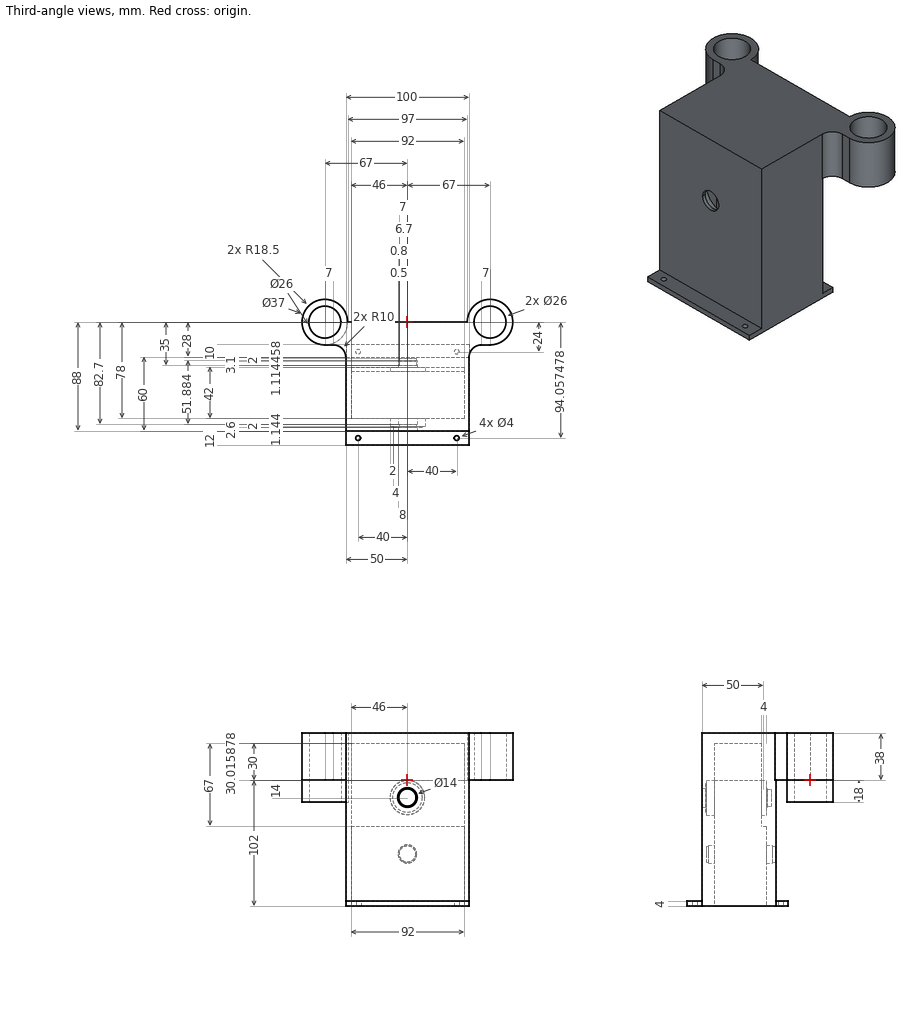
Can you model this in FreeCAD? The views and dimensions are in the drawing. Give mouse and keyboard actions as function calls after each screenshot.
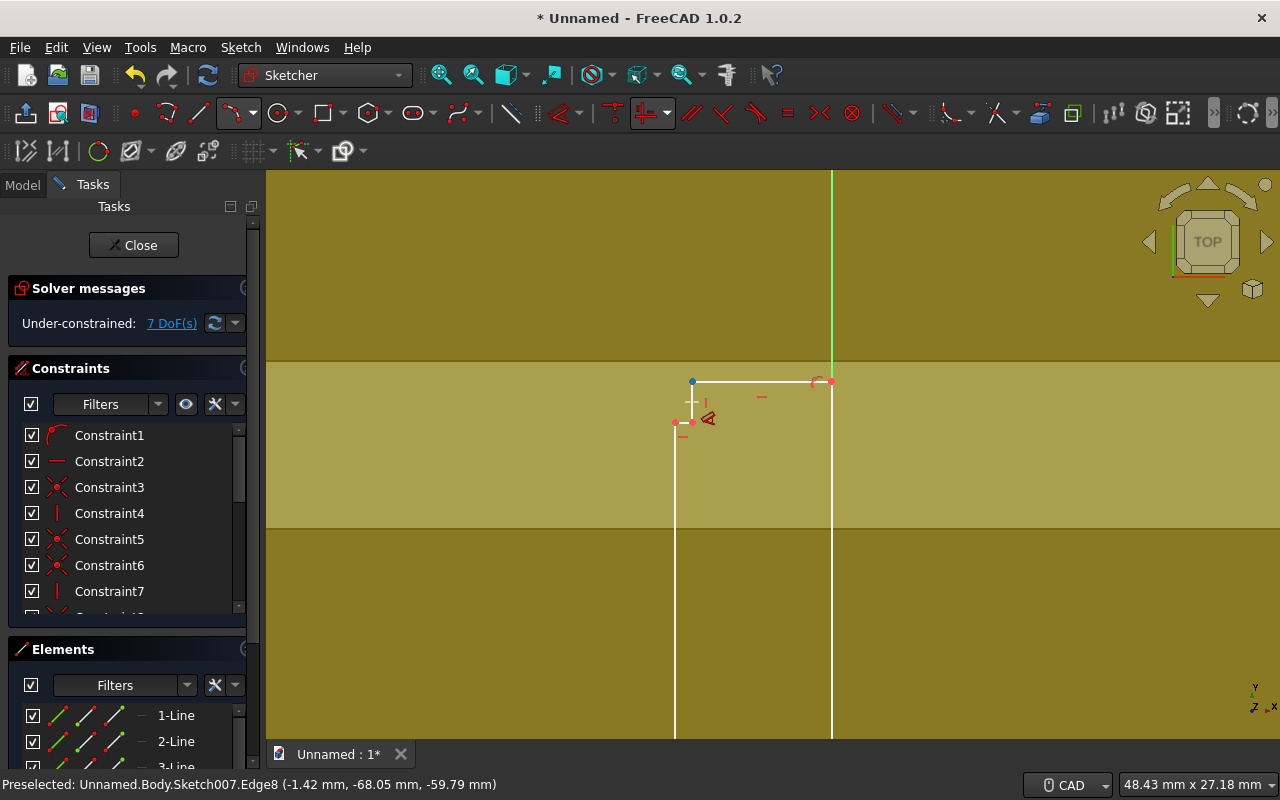
click(692, 402)
click(658, 402)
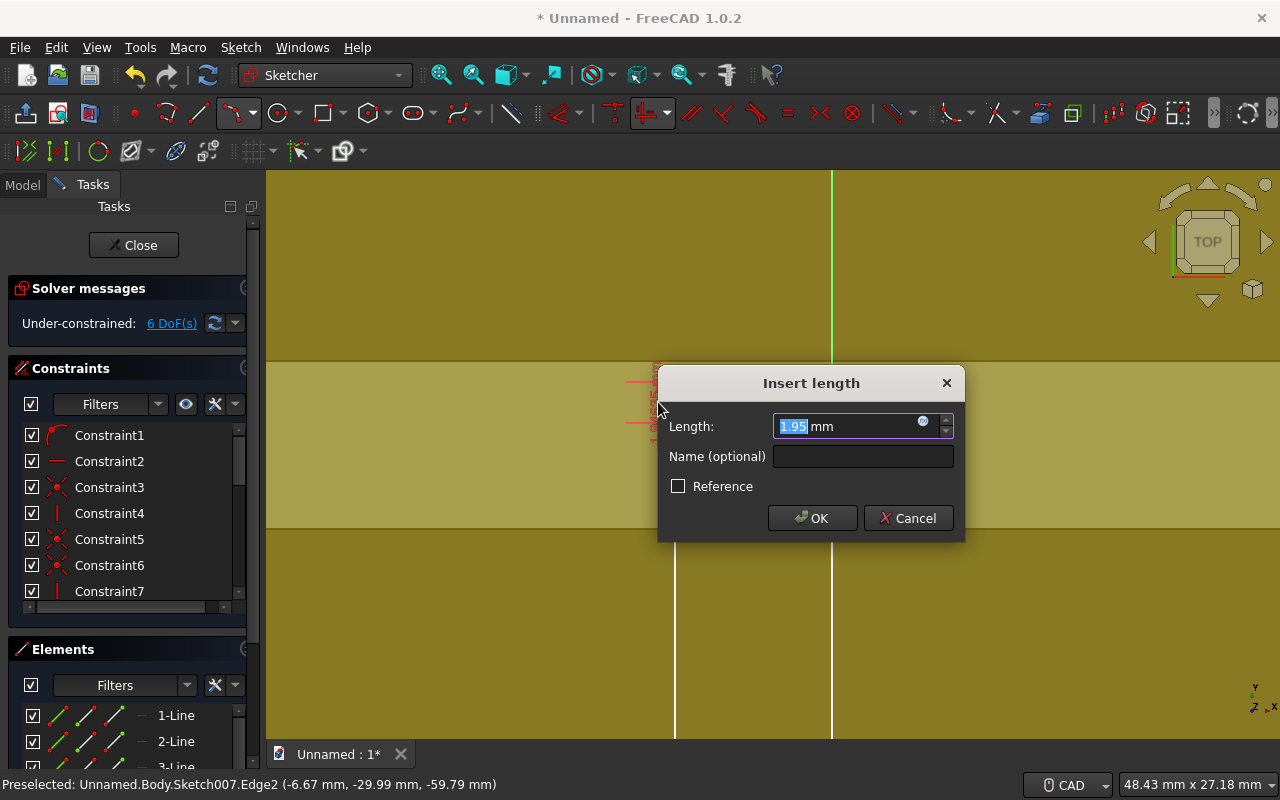
text(2)
key(Return)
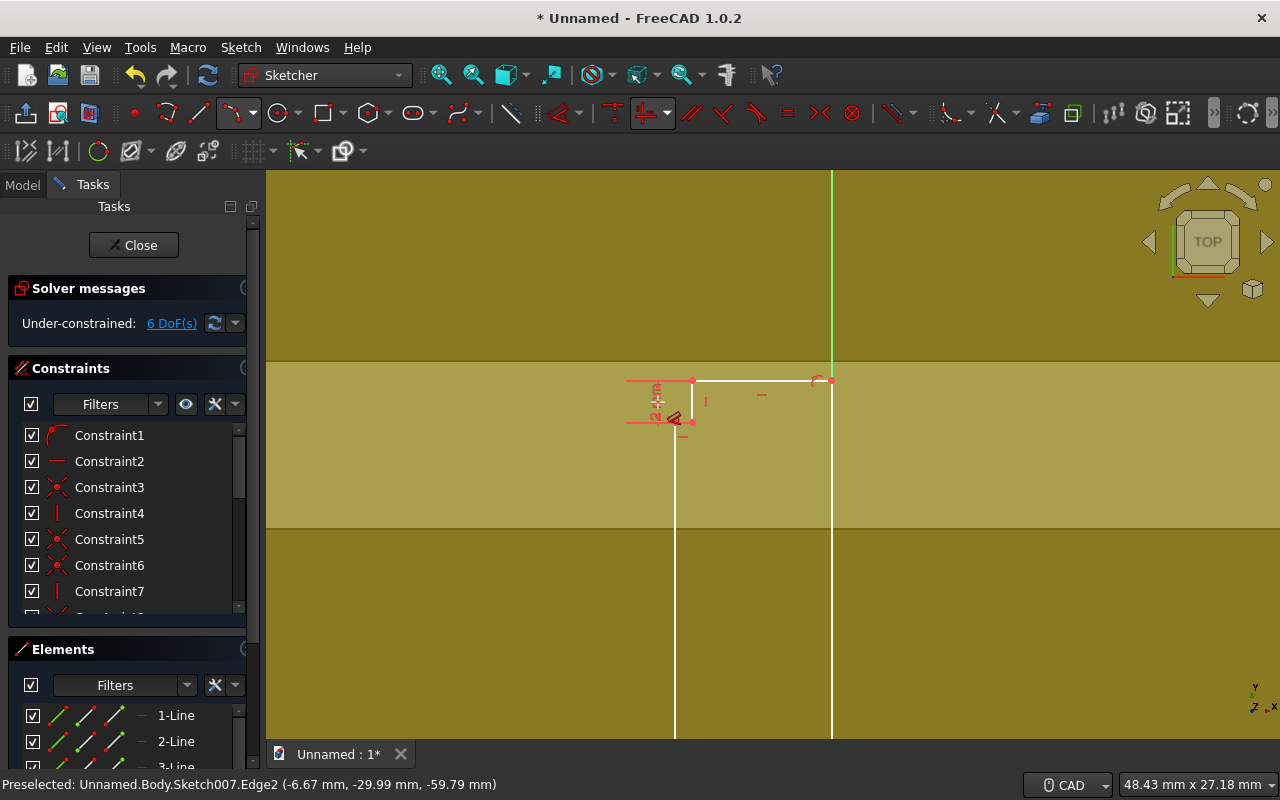
scroll(692, 402, down, 8)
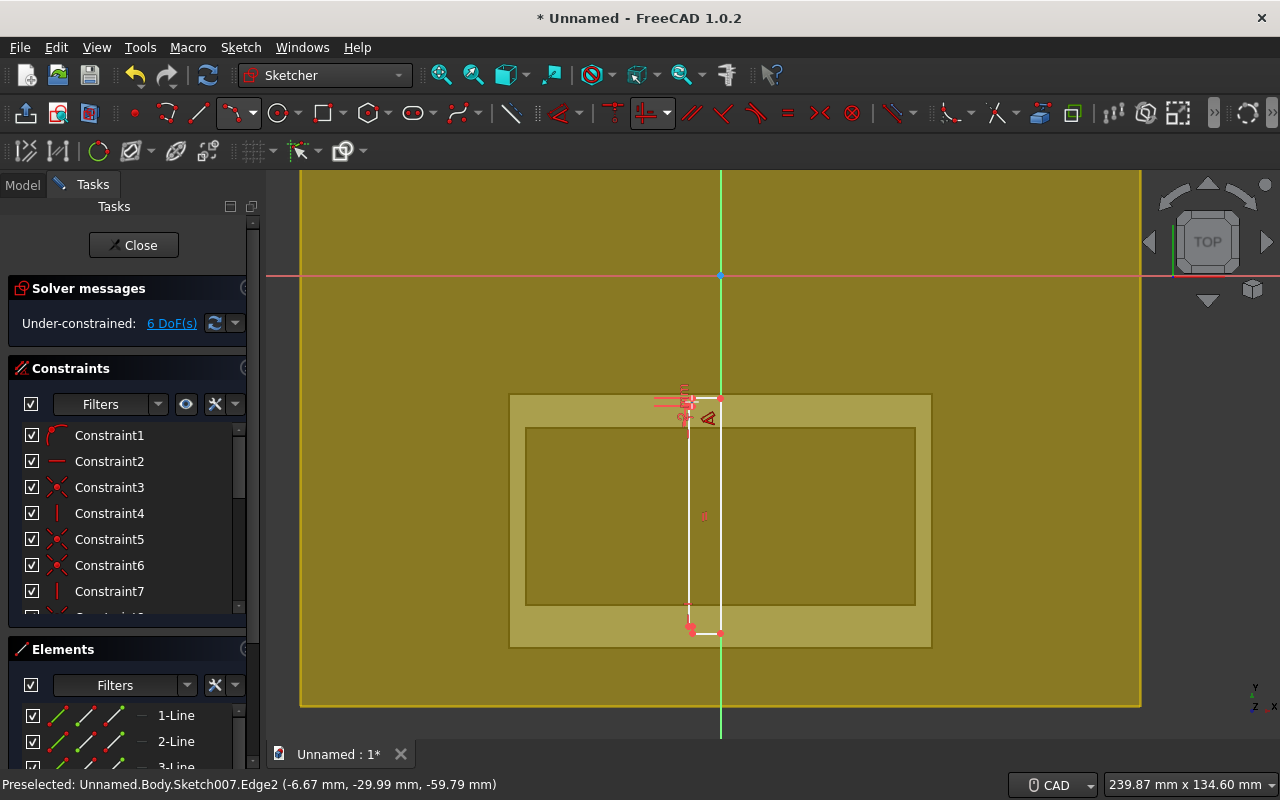
scroll(692, 629, up, 9)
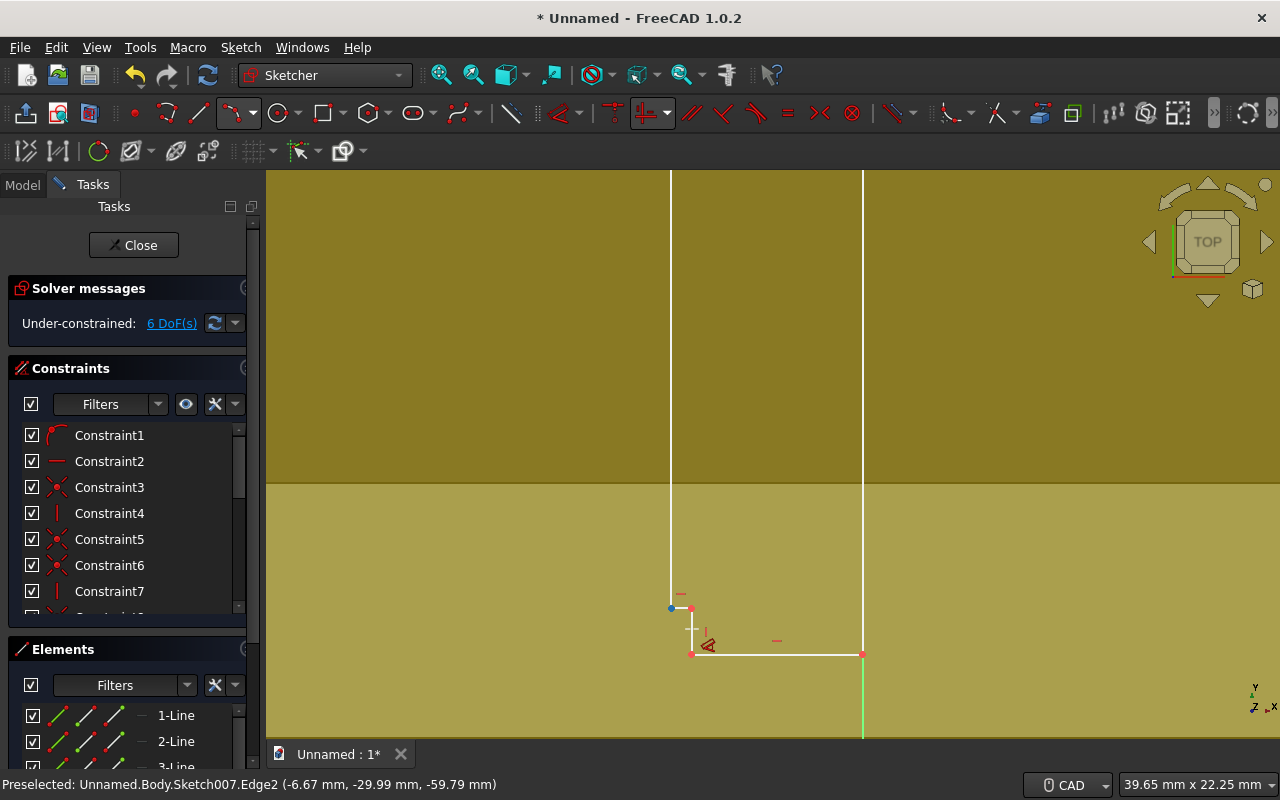
click(692, 622)
click(658, 631)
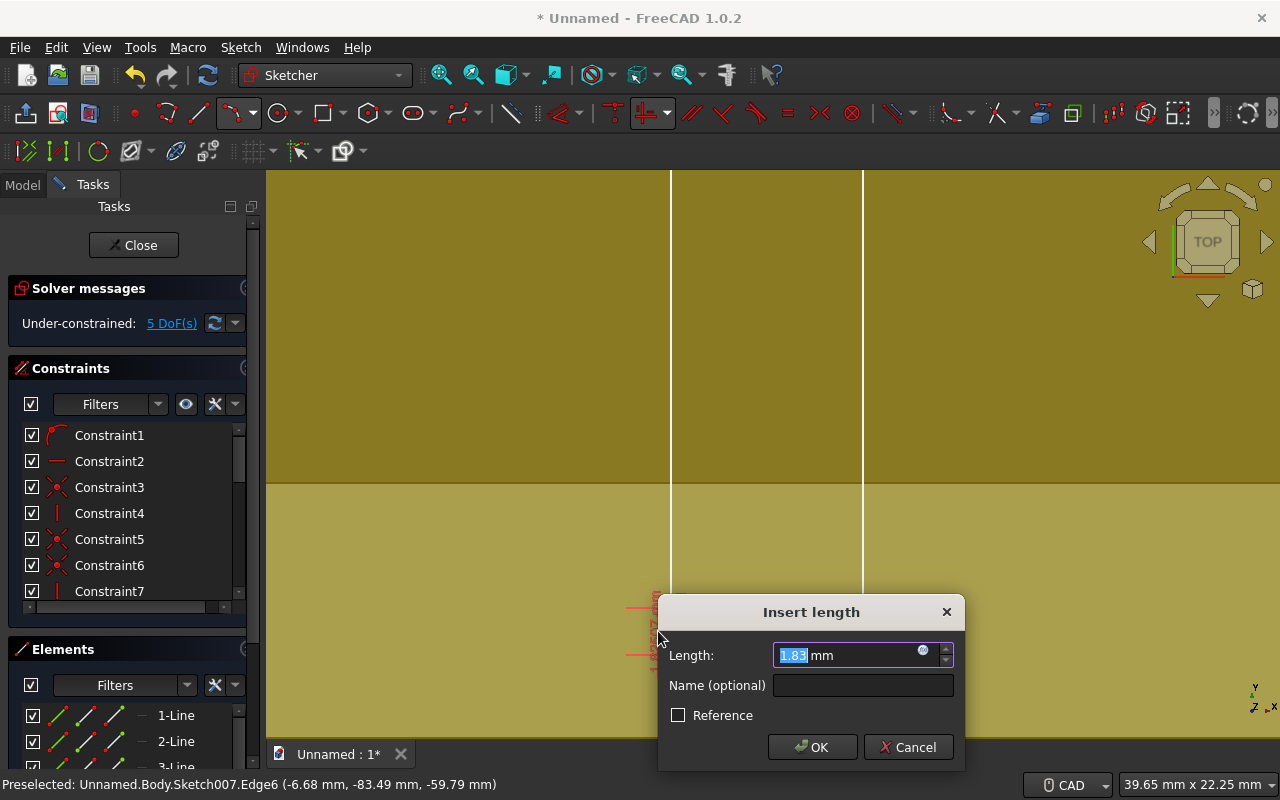
text(2)
key(Return)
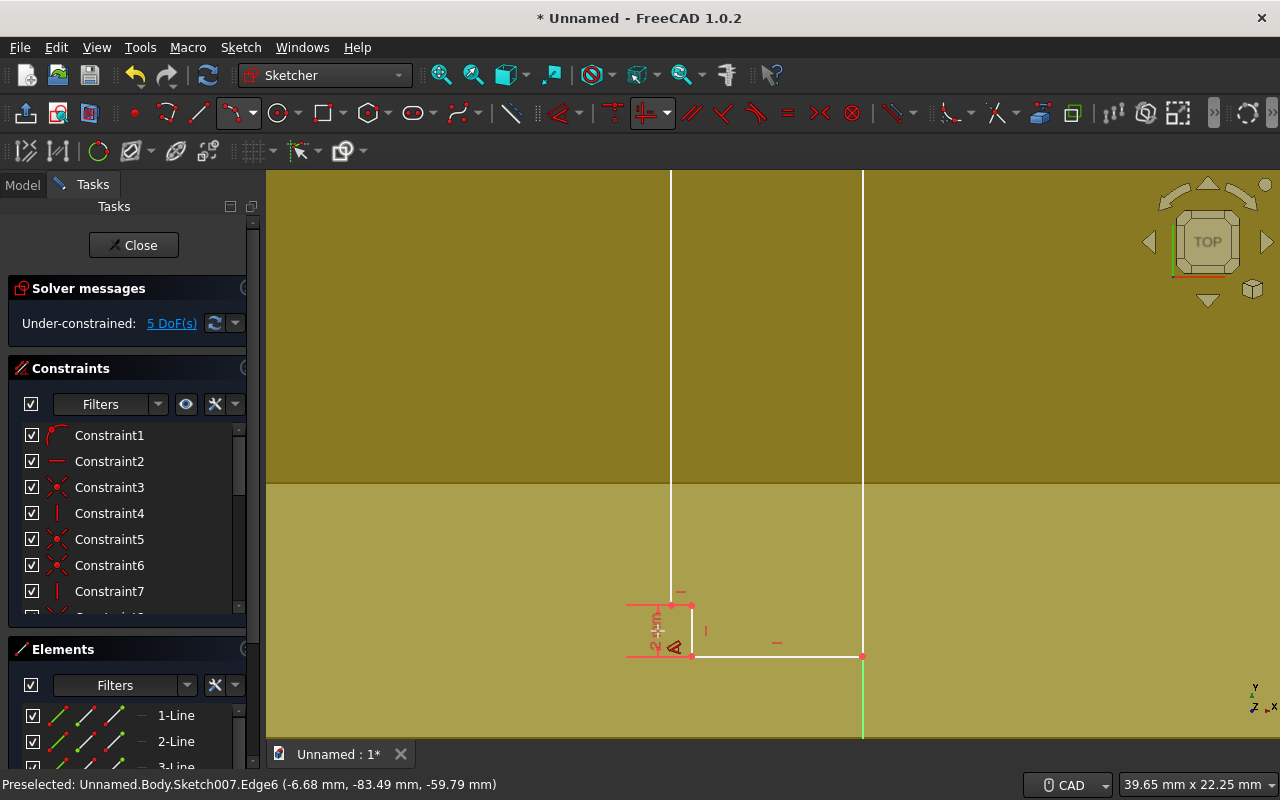
scroll(692, 629, down, 9)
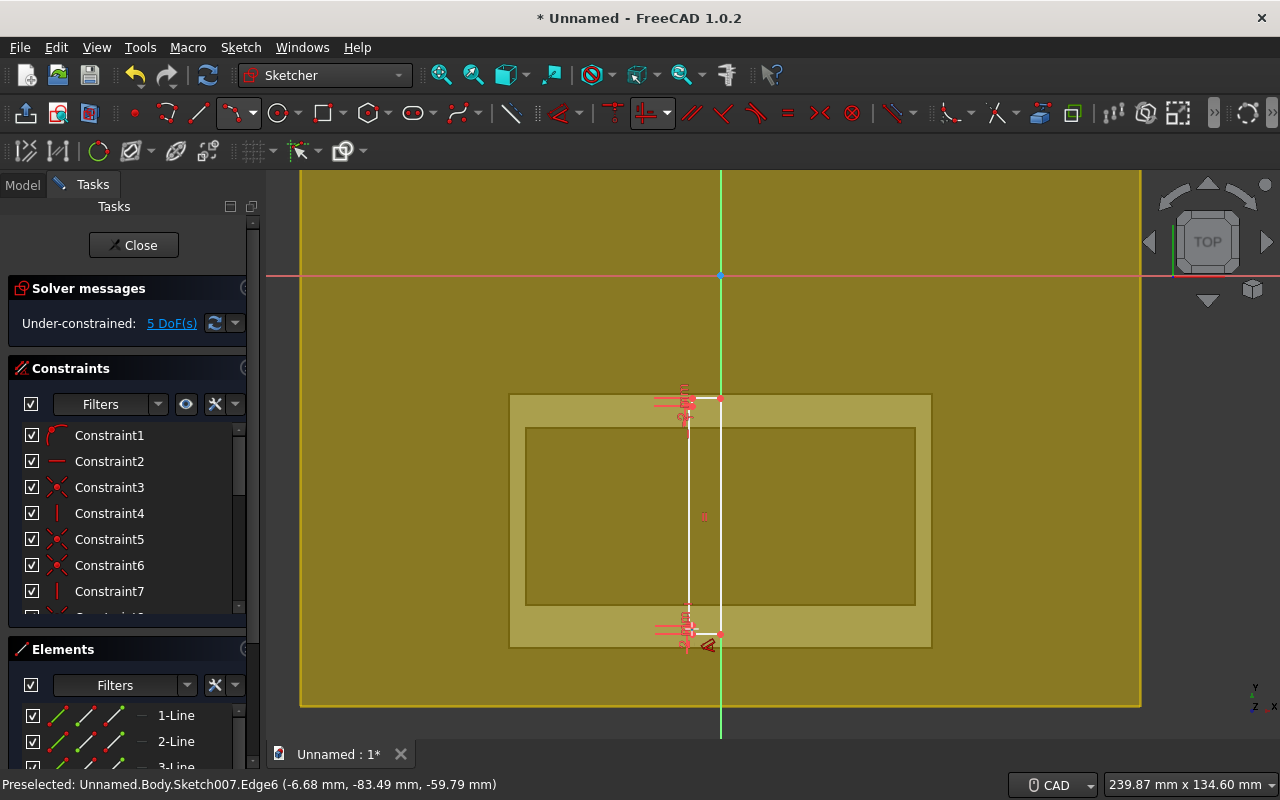
scroll(712, 398, up, 3)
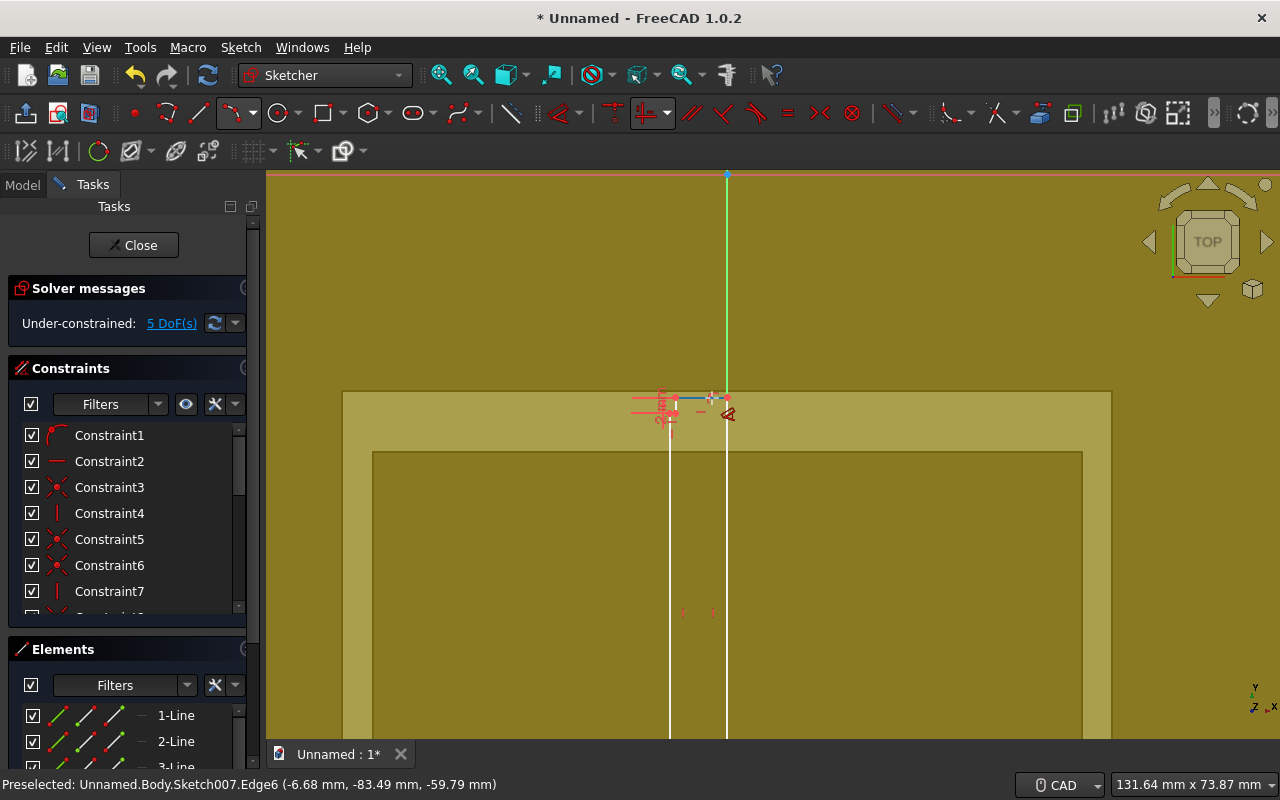
click(712, 398)
click(702, 364)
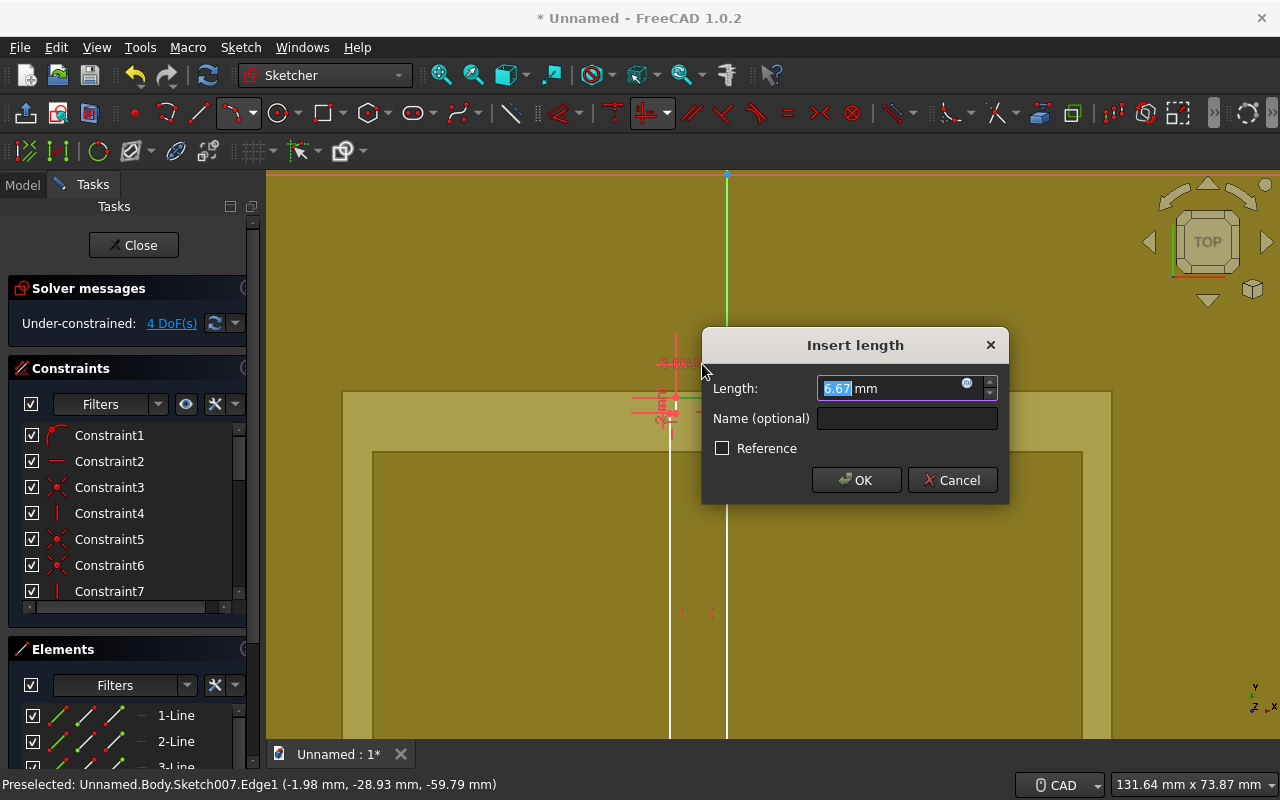
text(6.7)
key(Return)